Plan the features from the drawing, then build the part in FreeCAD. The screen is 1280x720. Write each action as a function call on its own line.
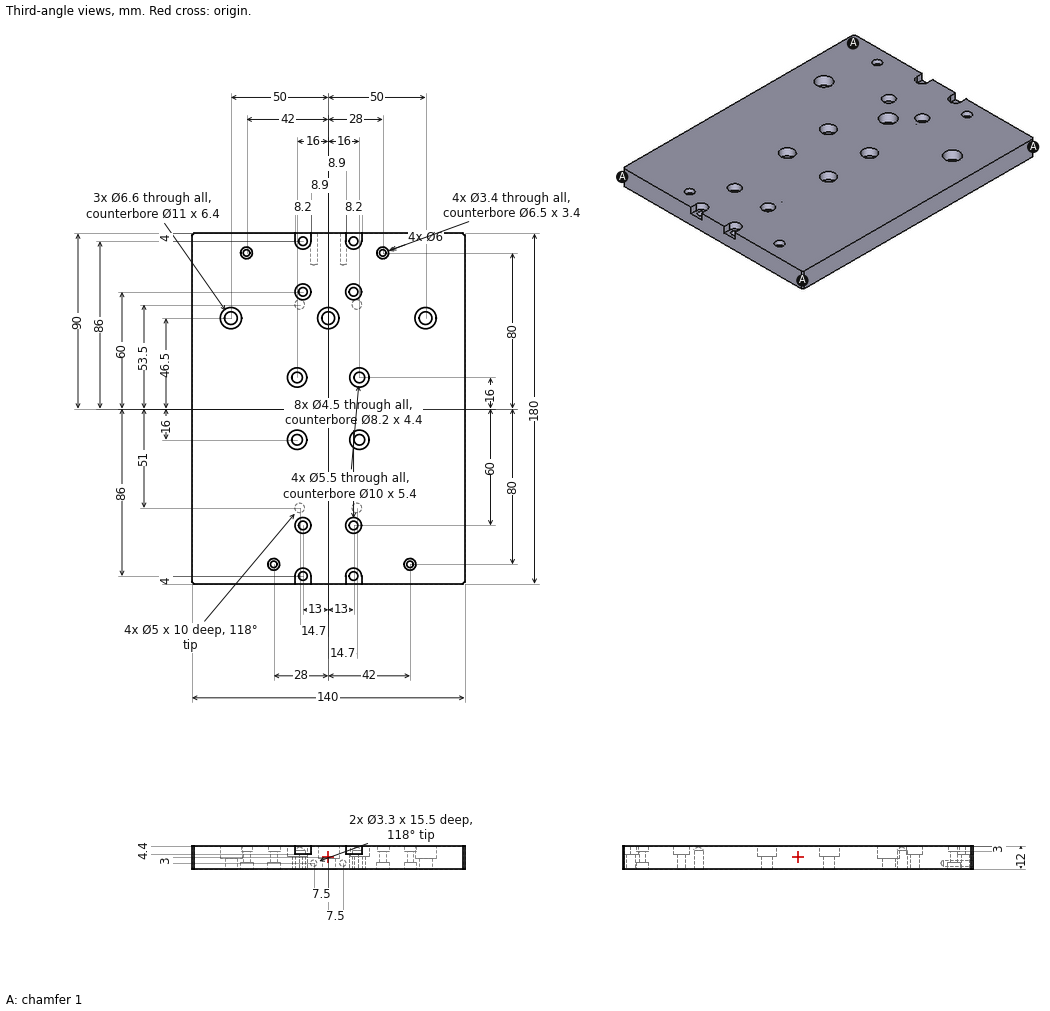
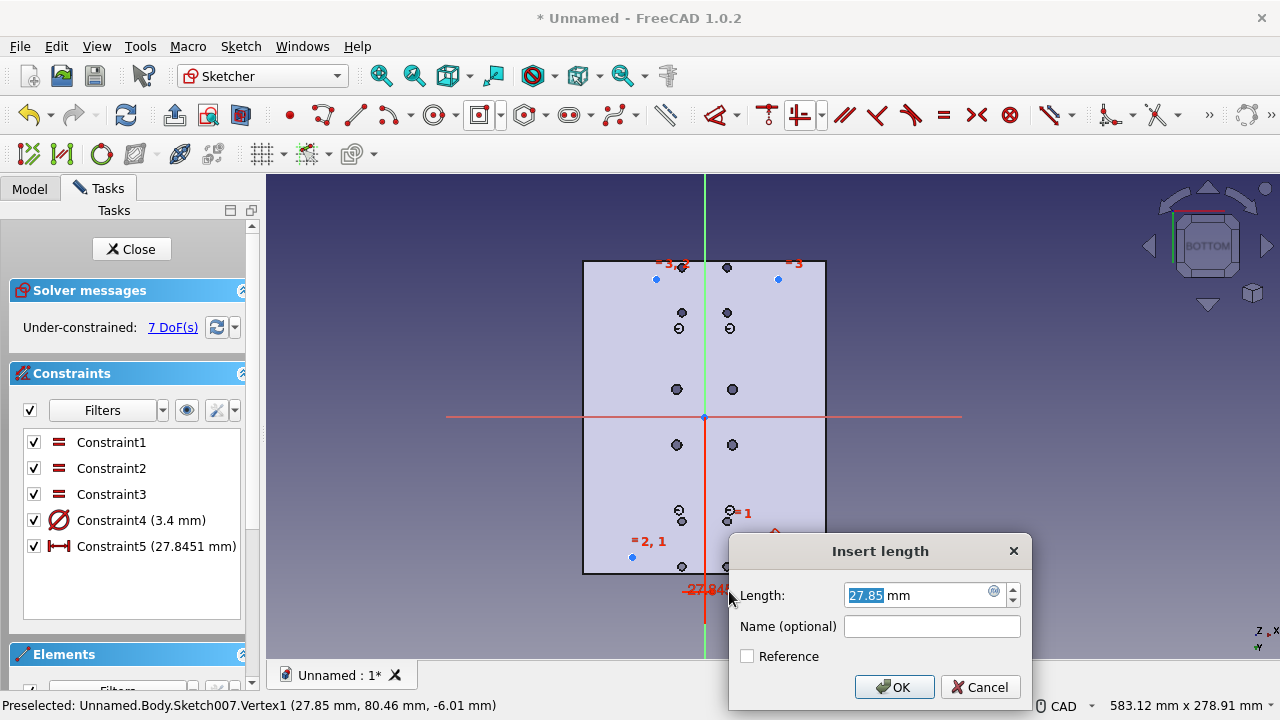
text(28)
key(Return)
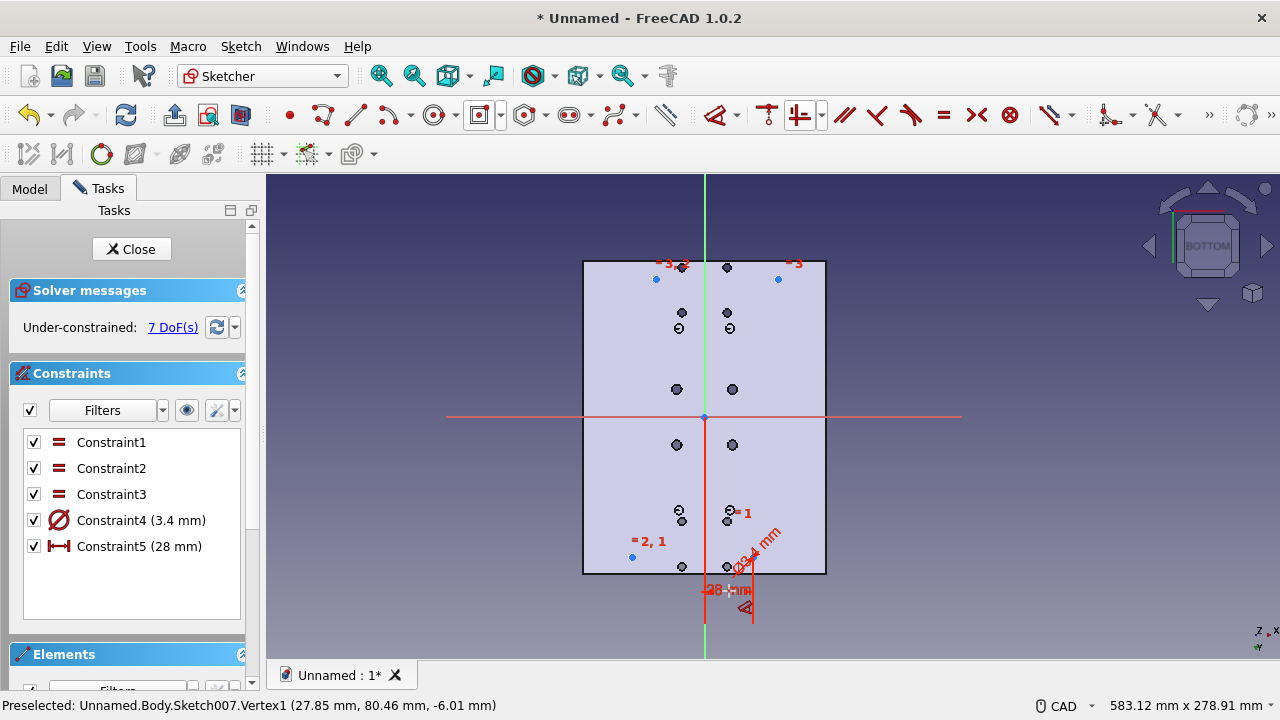
click(753, 557)
click(787, 487)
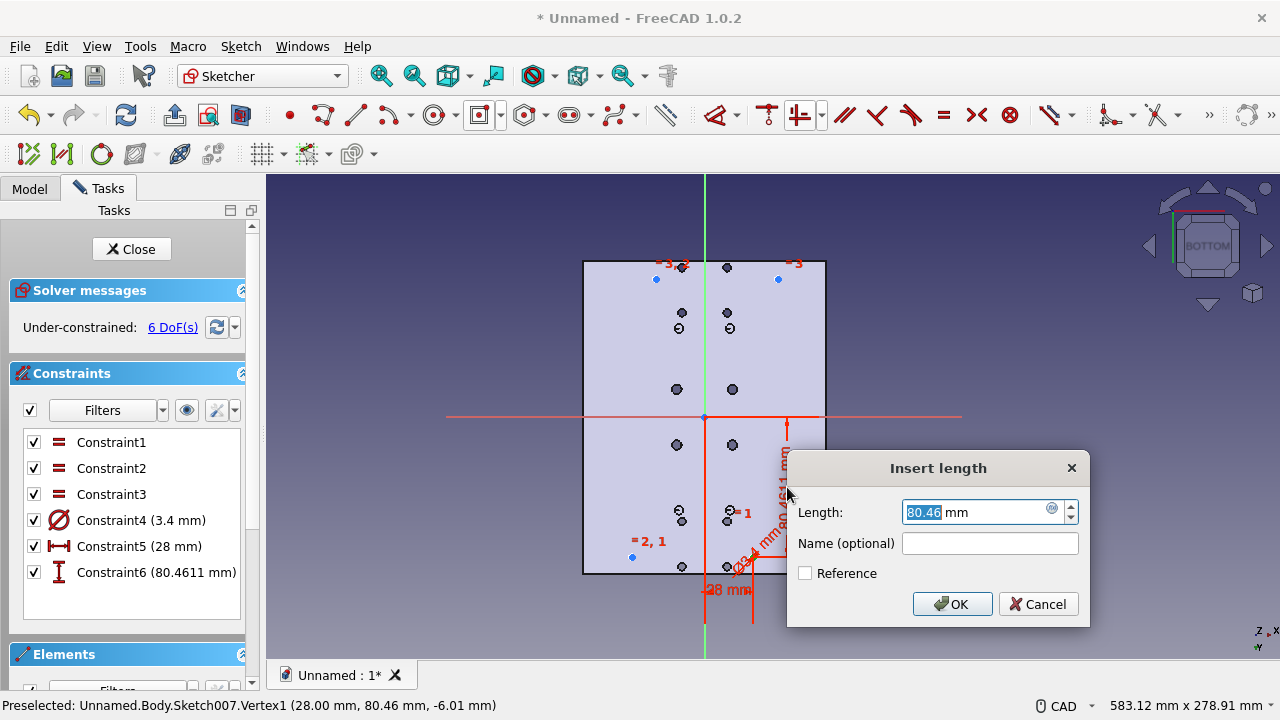
text(80)
key(Return)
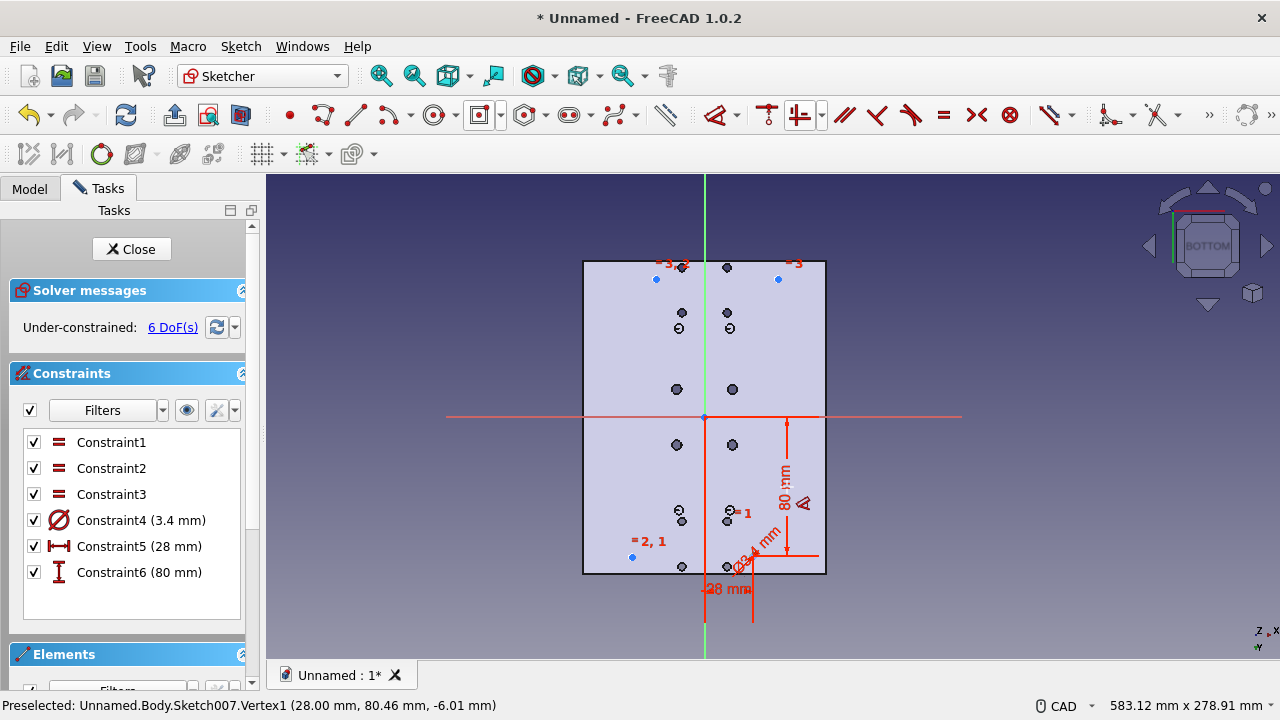
click(632, 557)
click(652, 591)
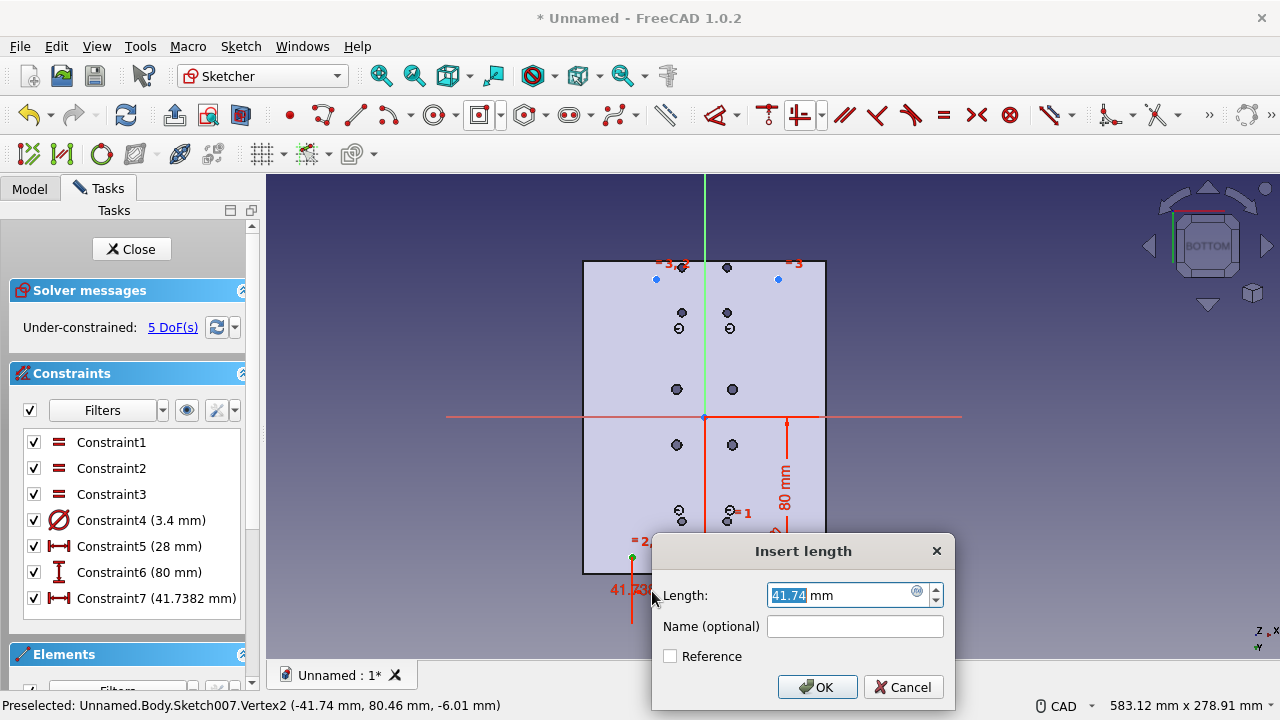
text(42)
key(Return)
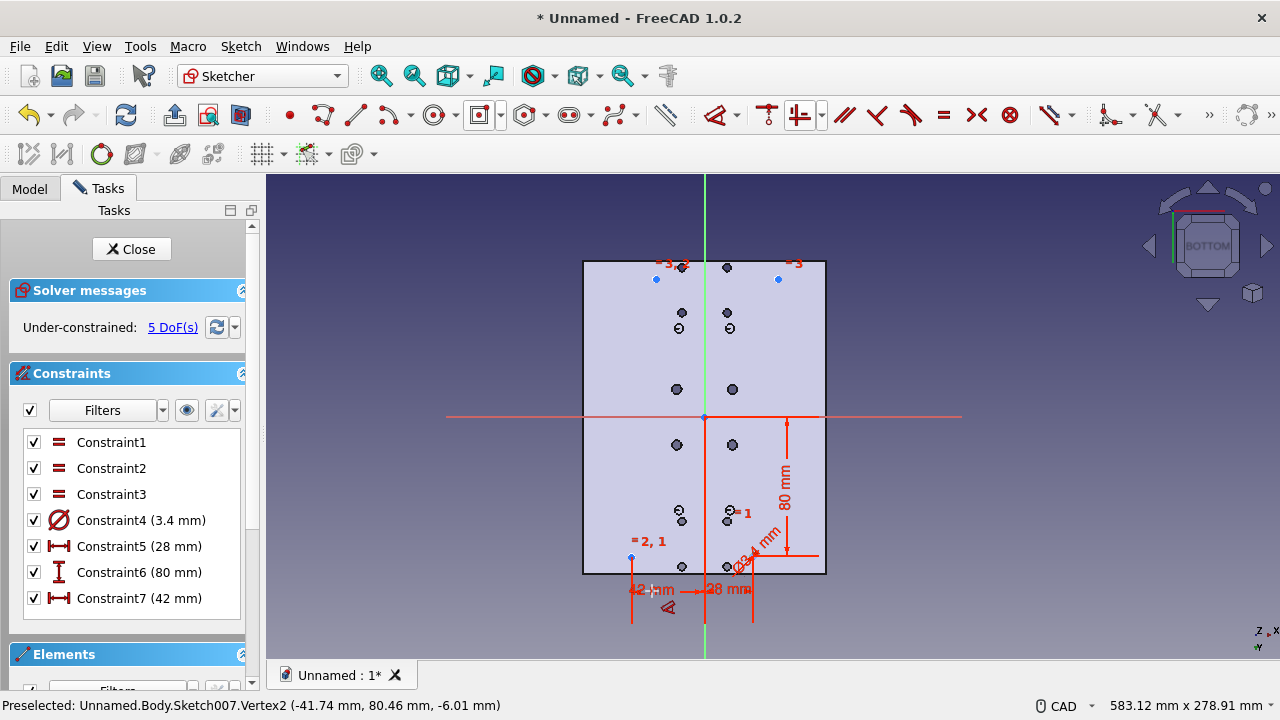
click(632, 557)
click(598, 487)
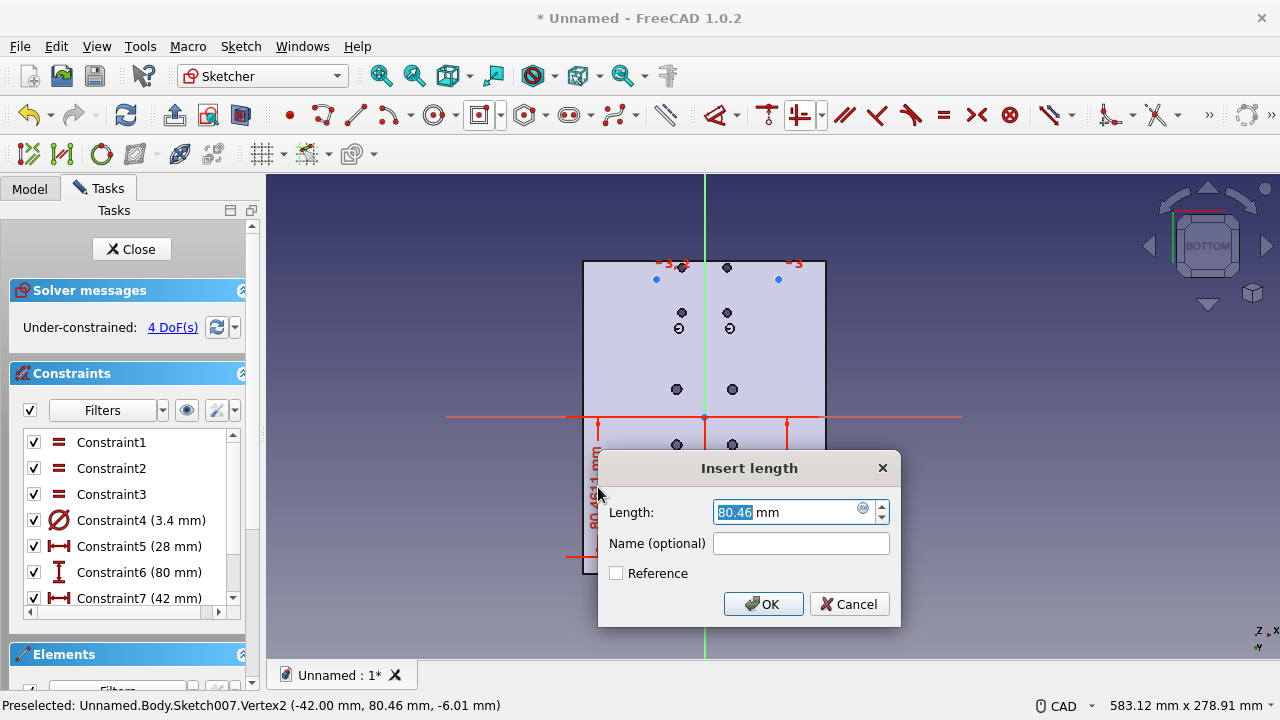
text(80)
key(Return)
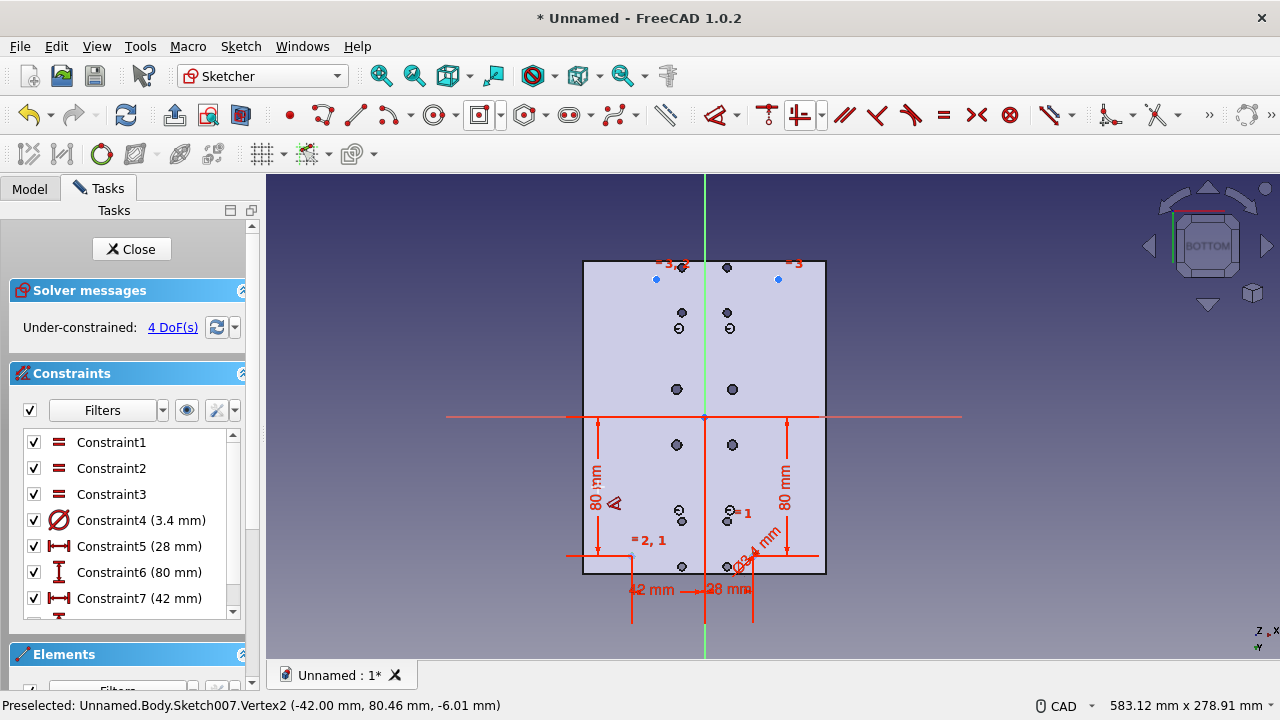
click(656, 279)
click(680, 245)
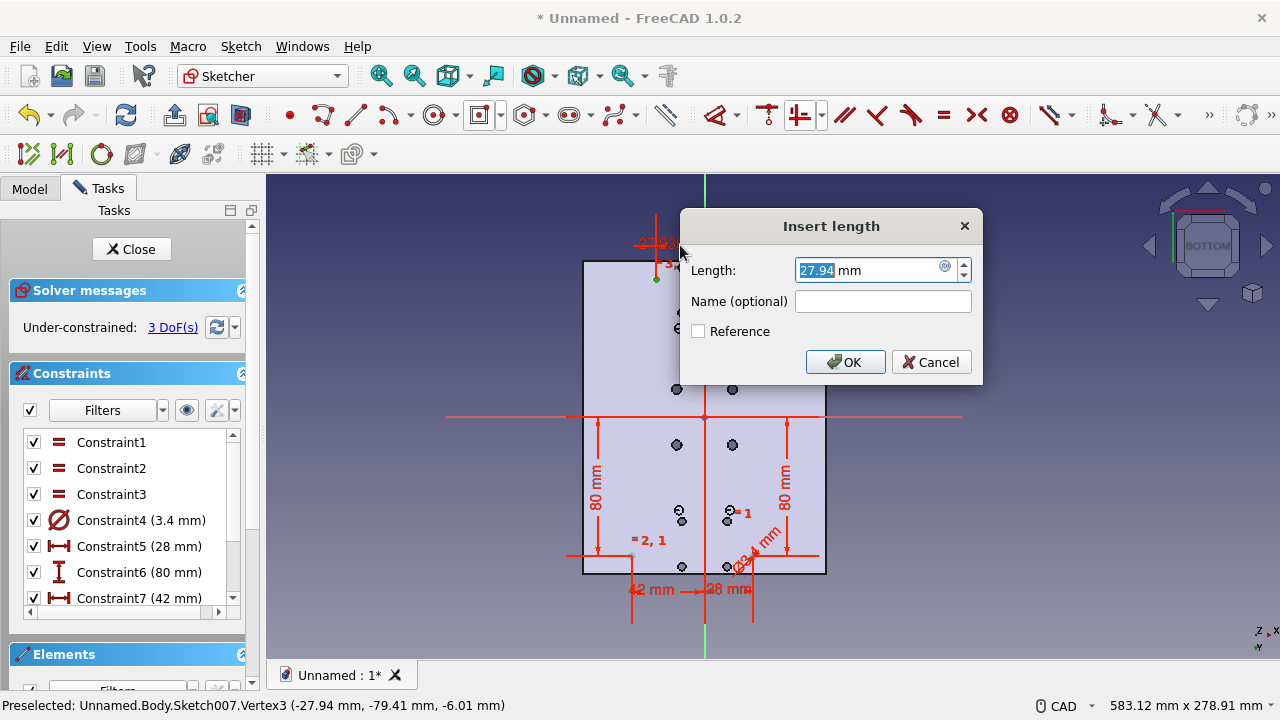
text(28)
key(Return)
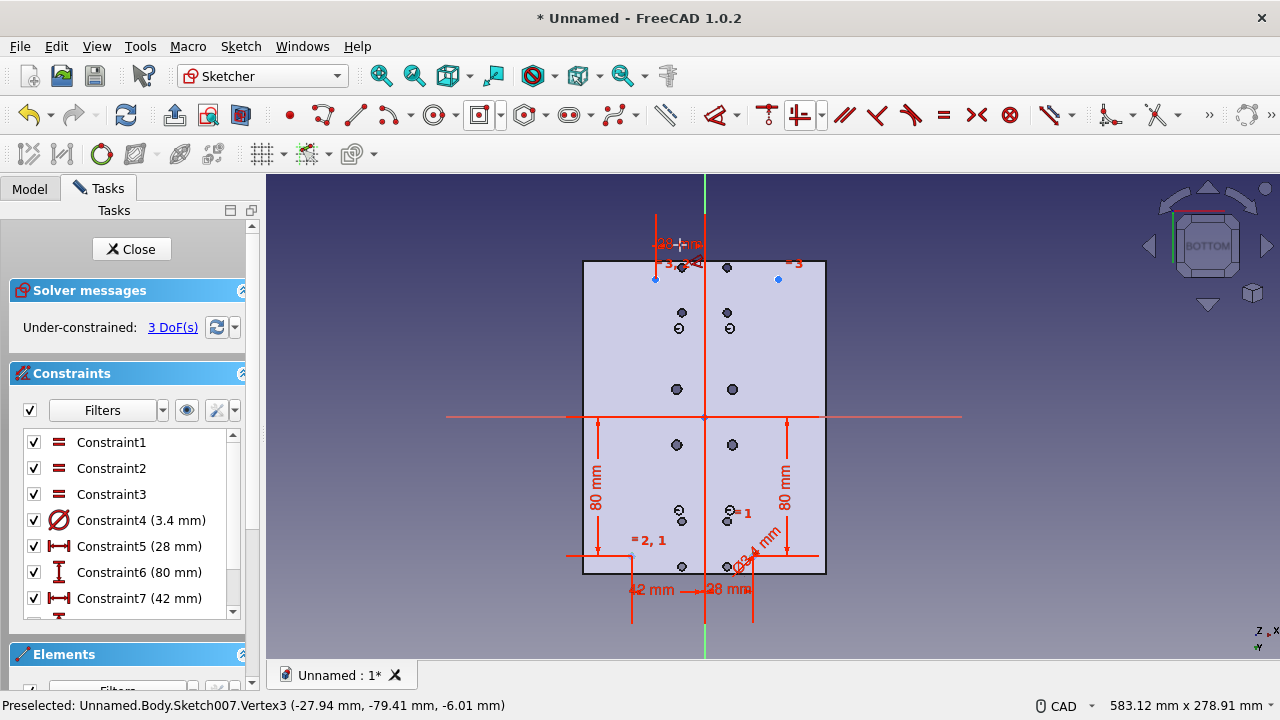
click(656, 279)
click(622, 348)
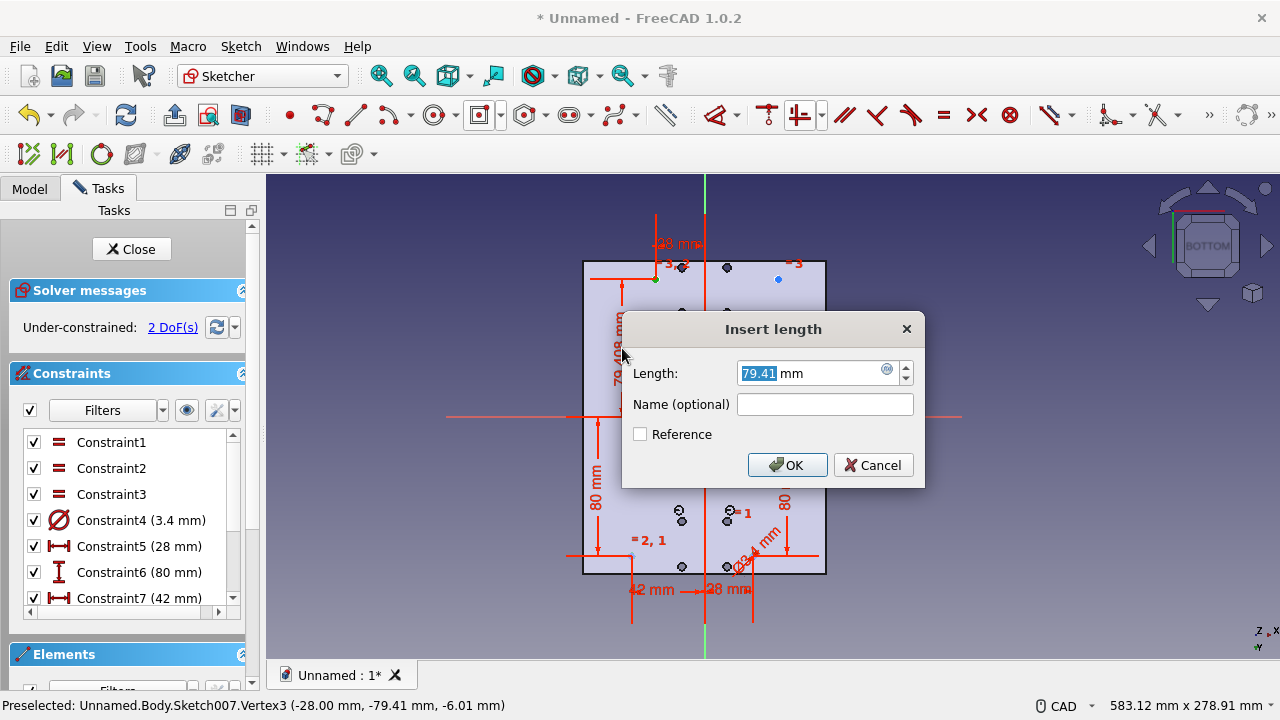
text(80)
key(Return)